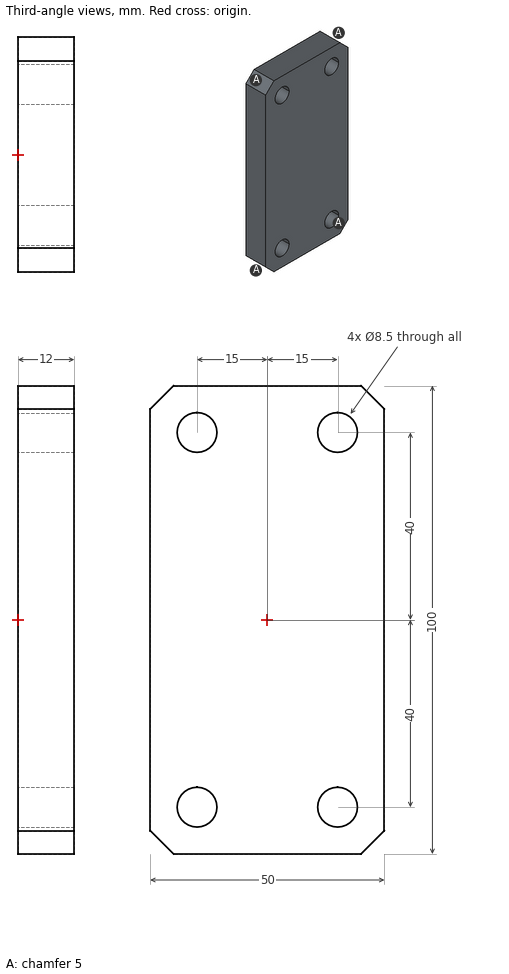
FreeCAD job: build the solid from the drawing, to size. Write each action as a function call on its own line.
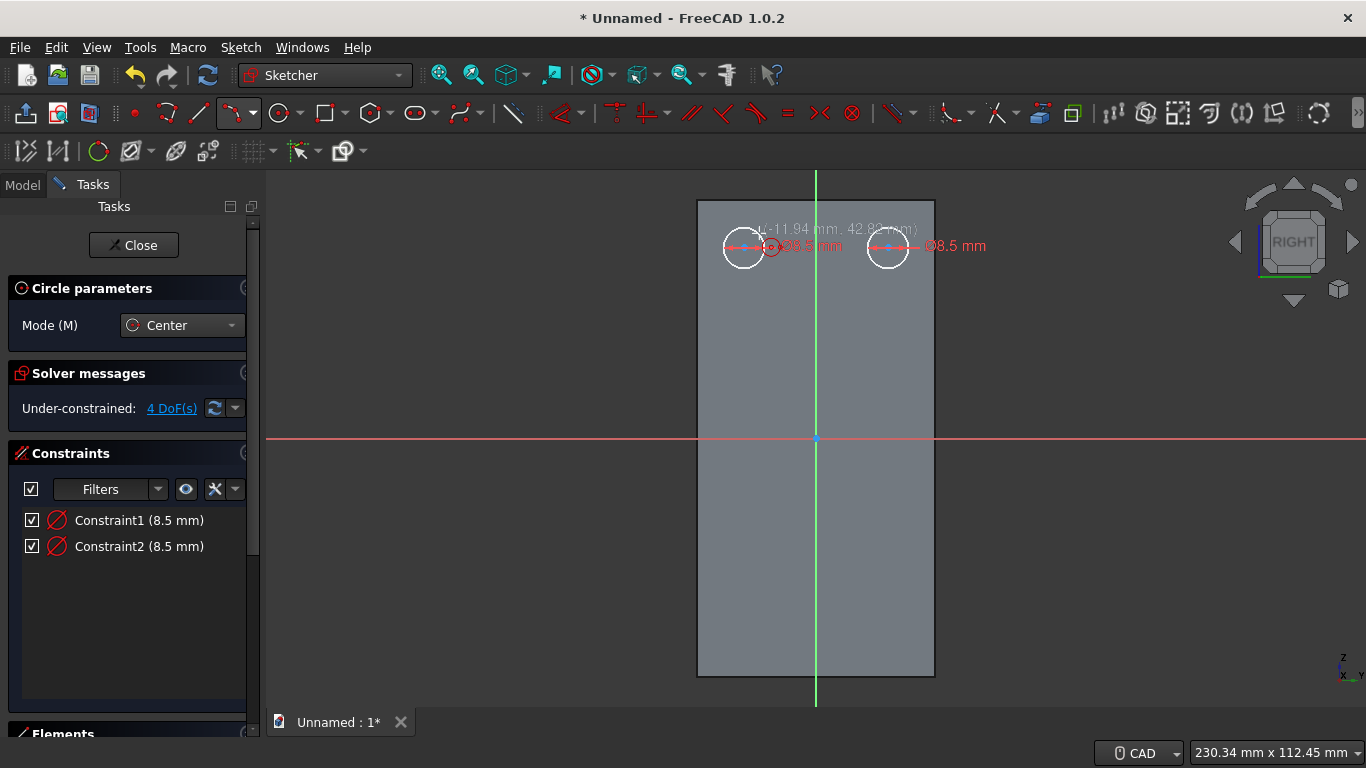
click(888, 630)
move(902, 615)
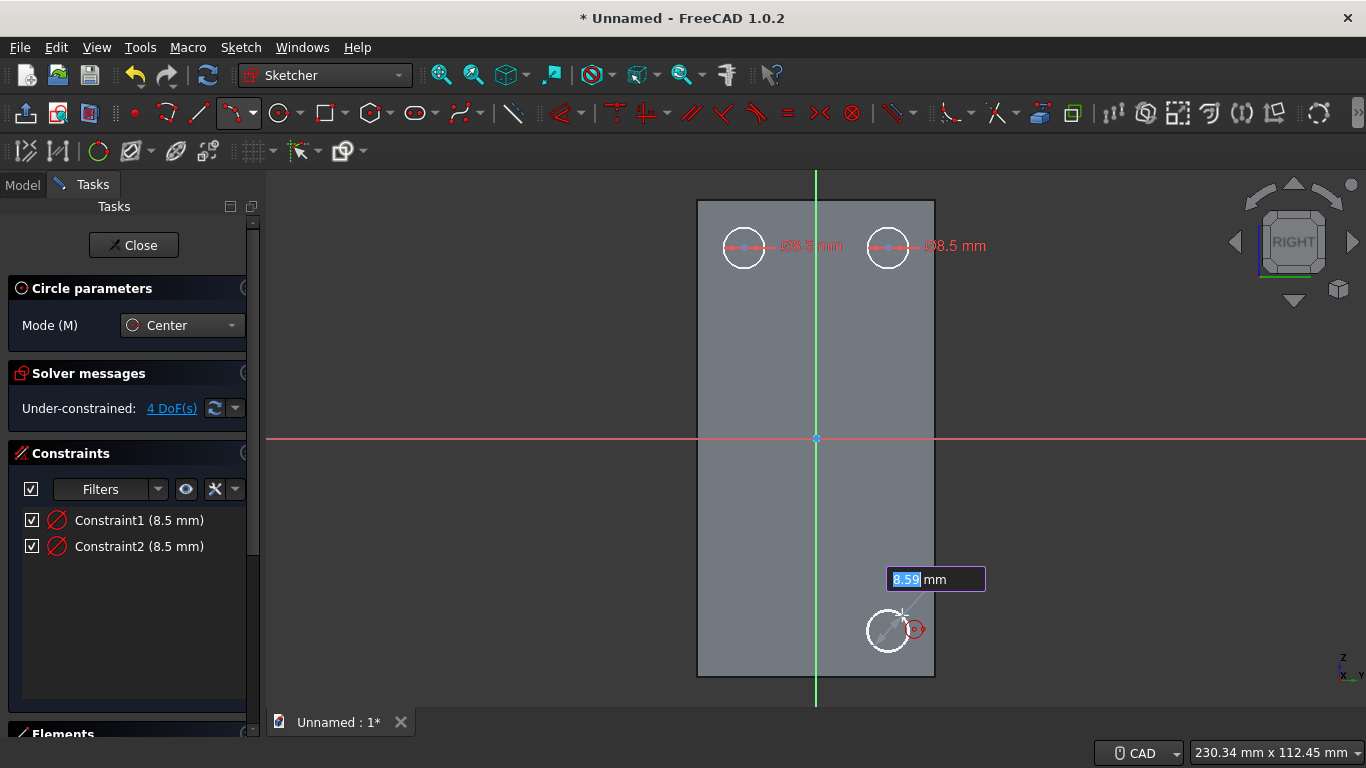
text(8.5)
key(Return)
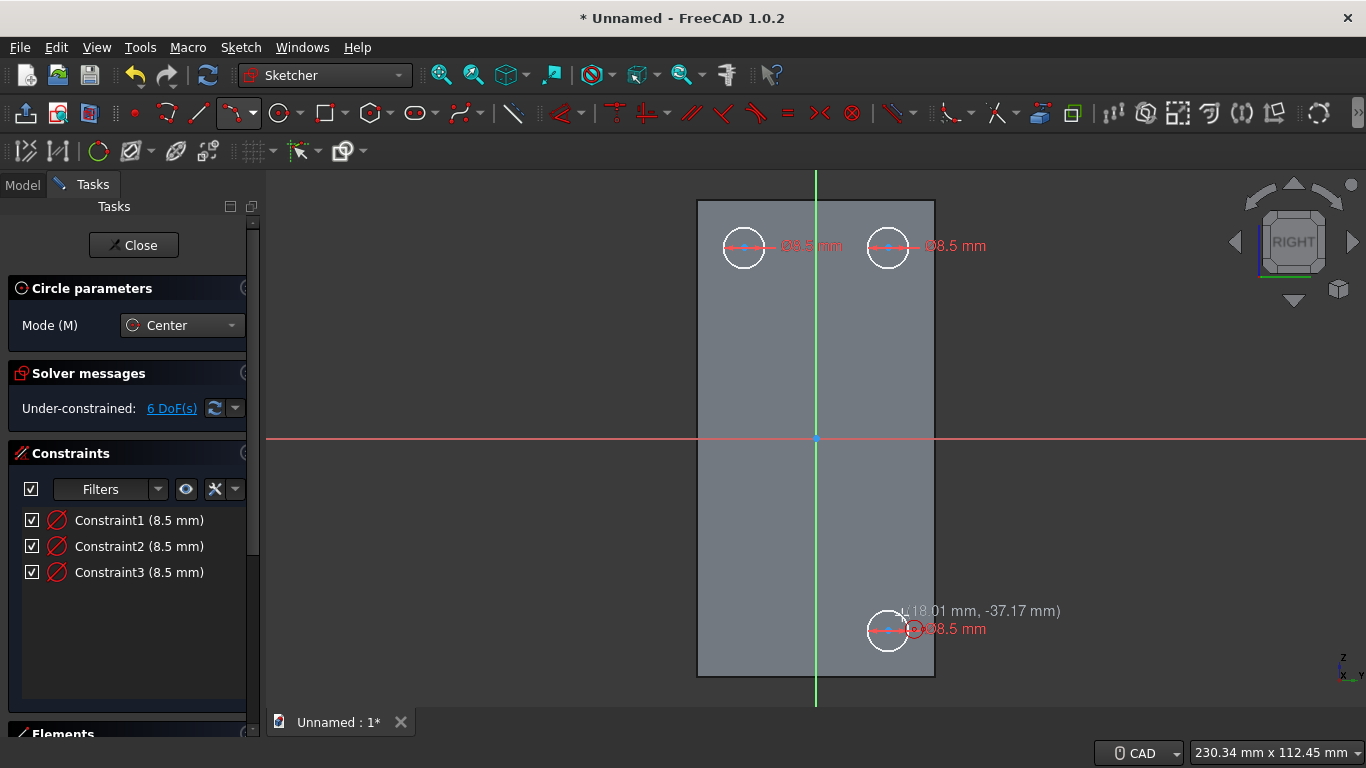
click(744, 630)
move(759, 615)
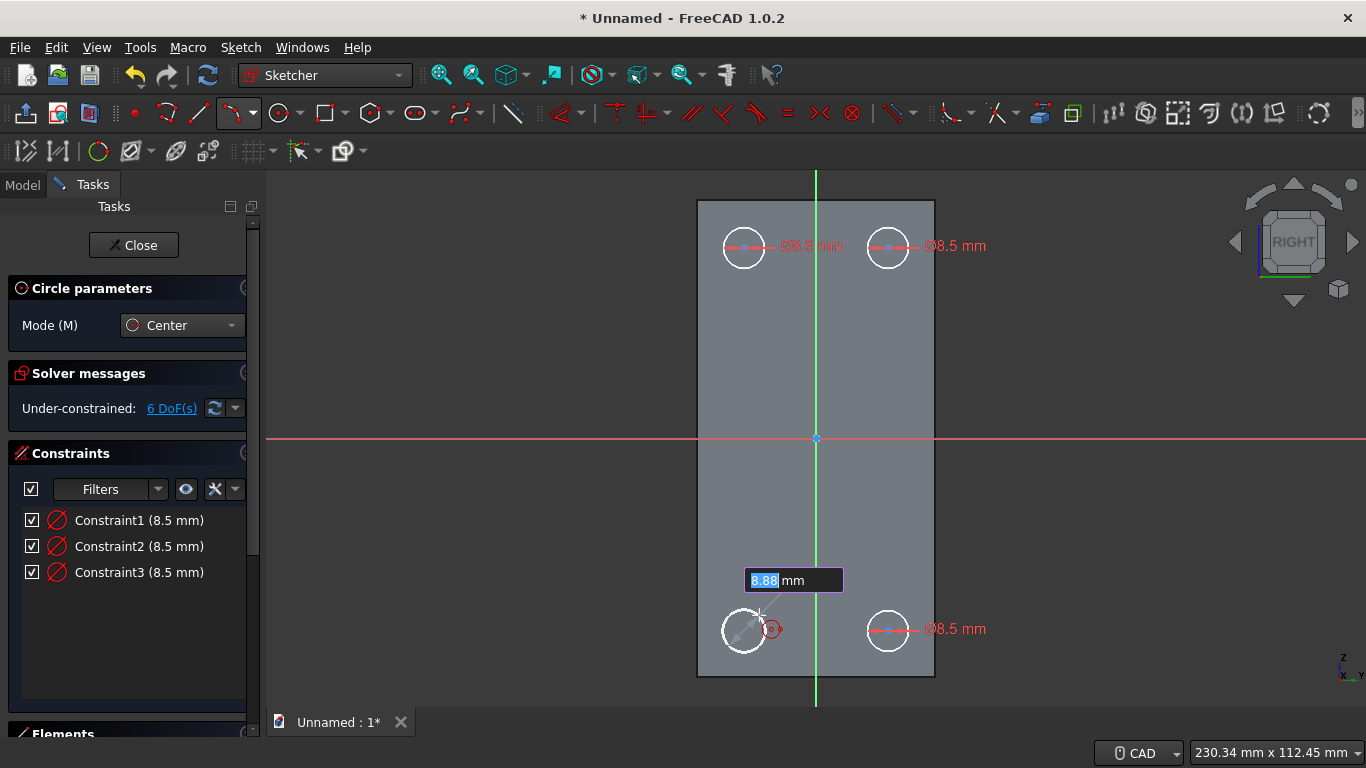
text(8.5)
key(Return)
key(Escape)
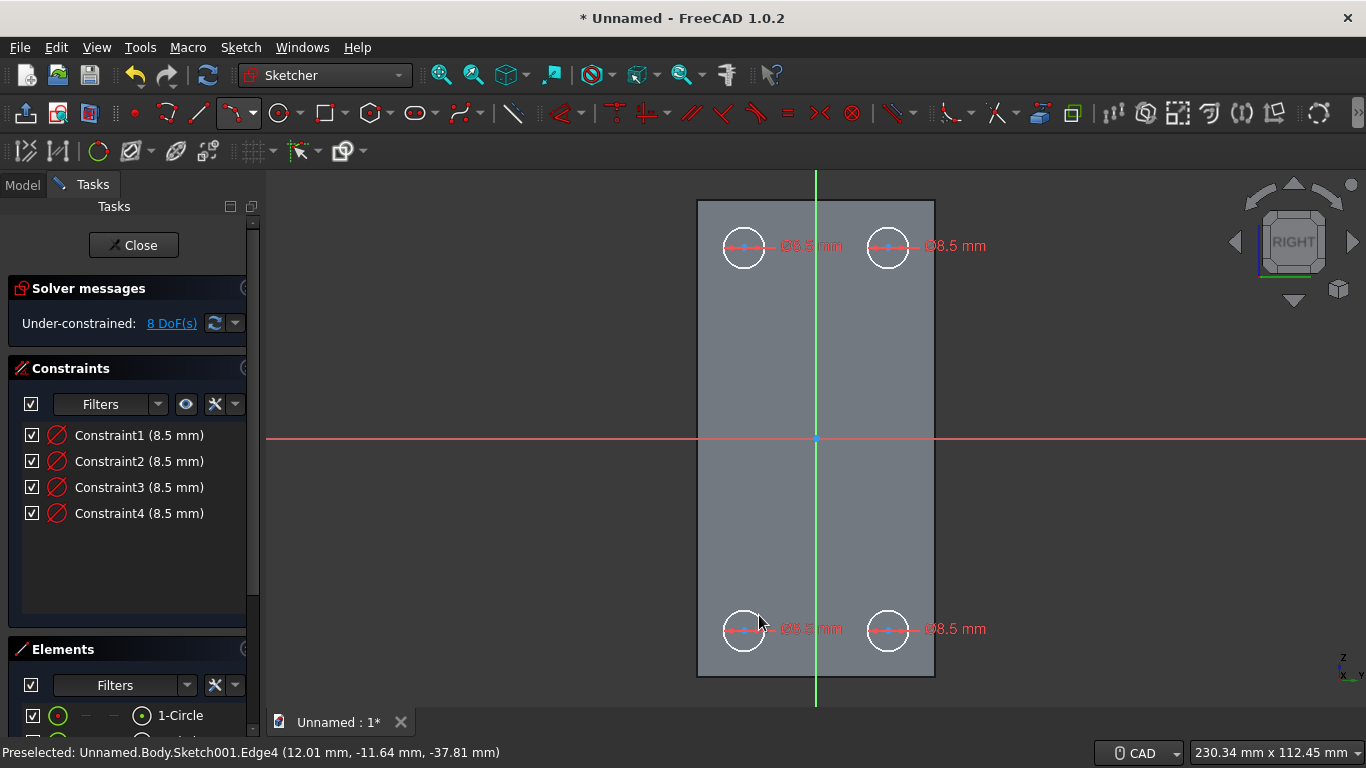
click(888, 248)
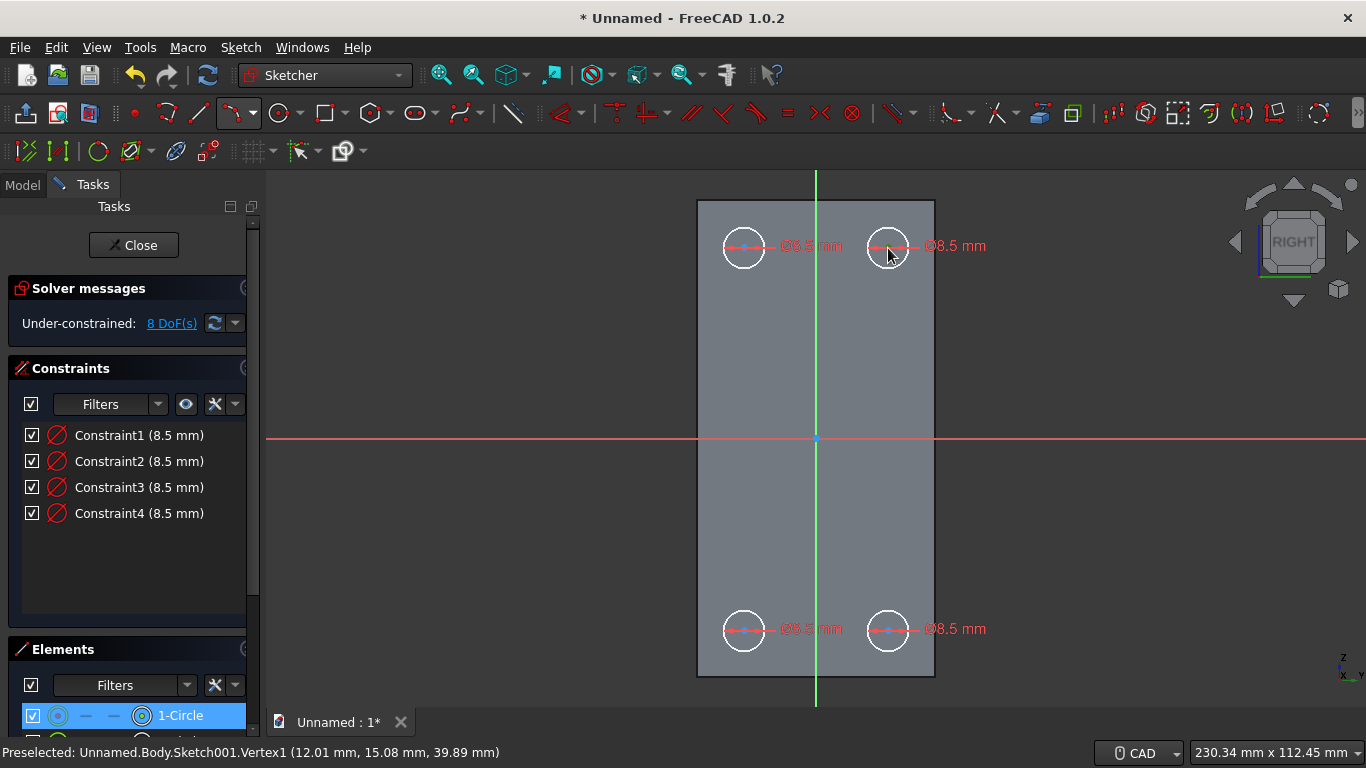
click(744, 248)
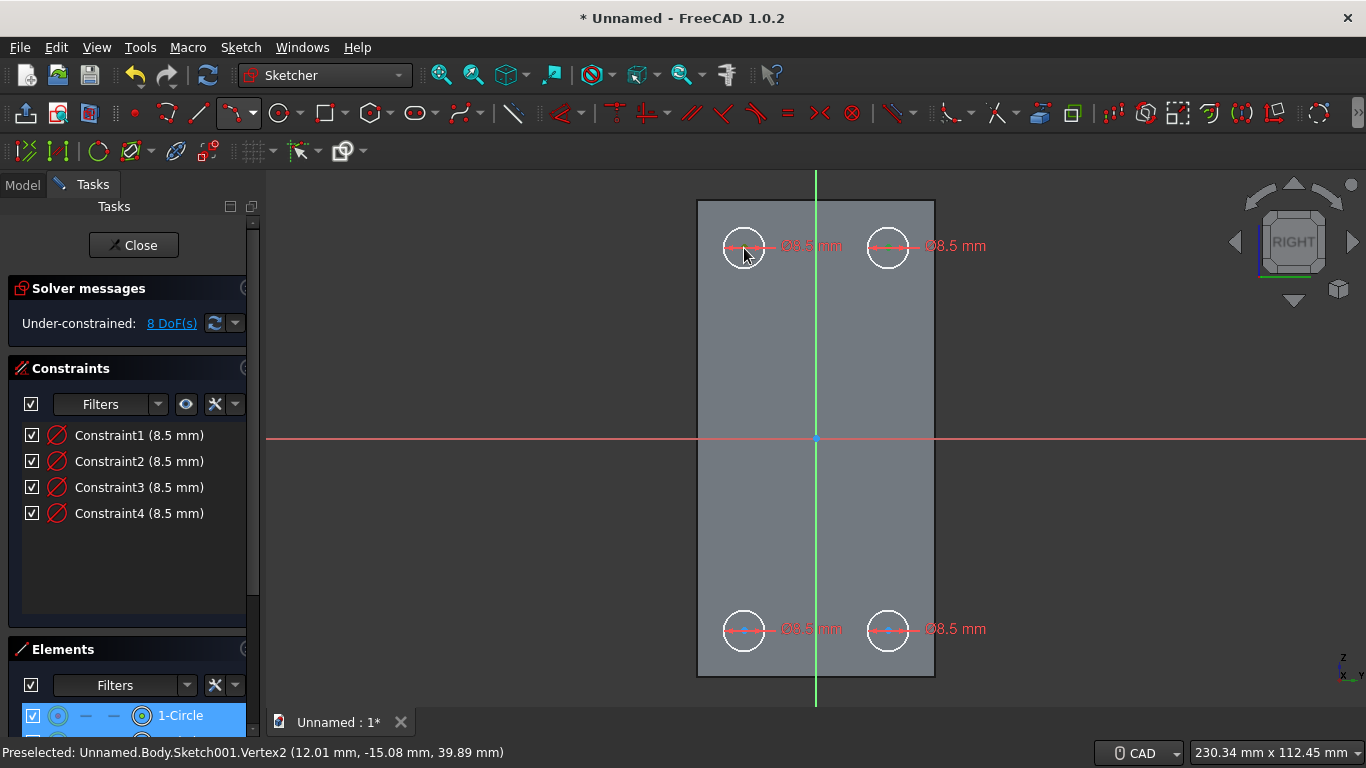
click(670, 114)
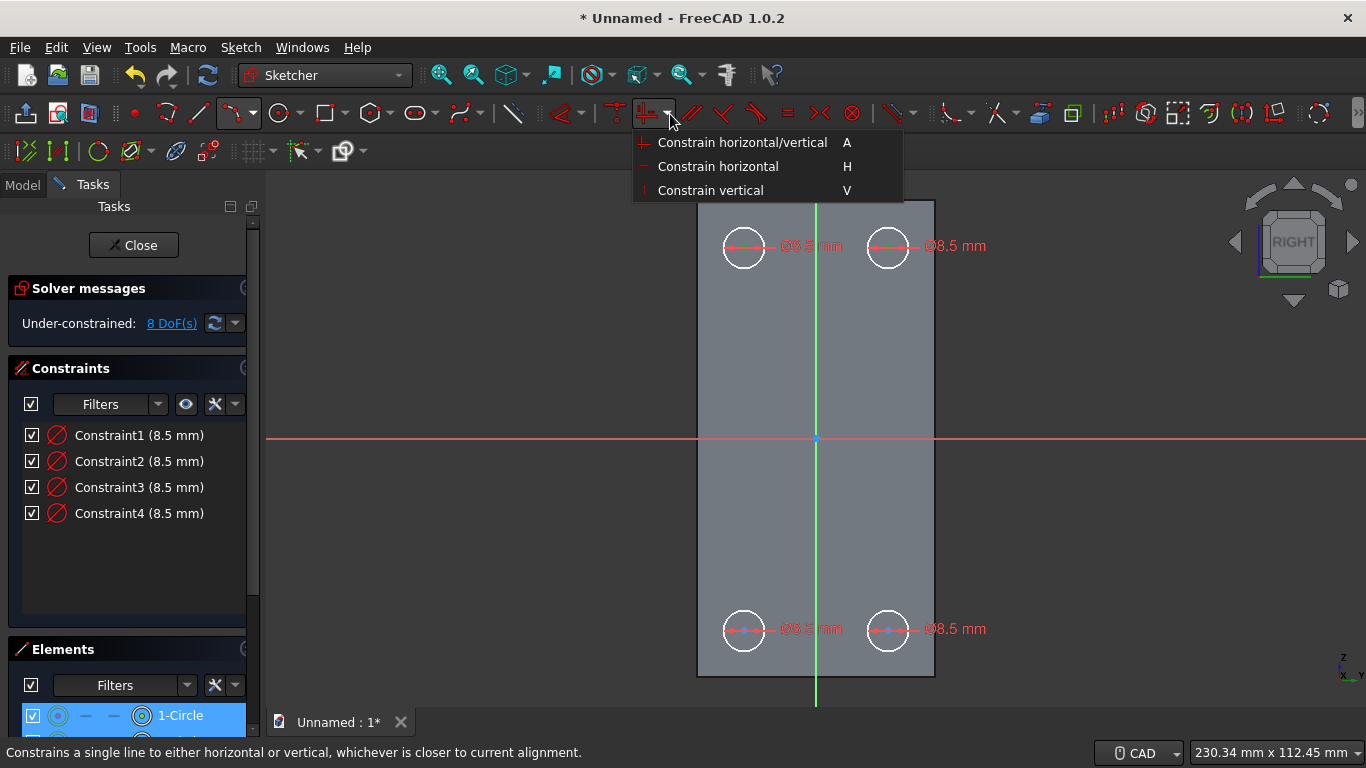
click(768, 166)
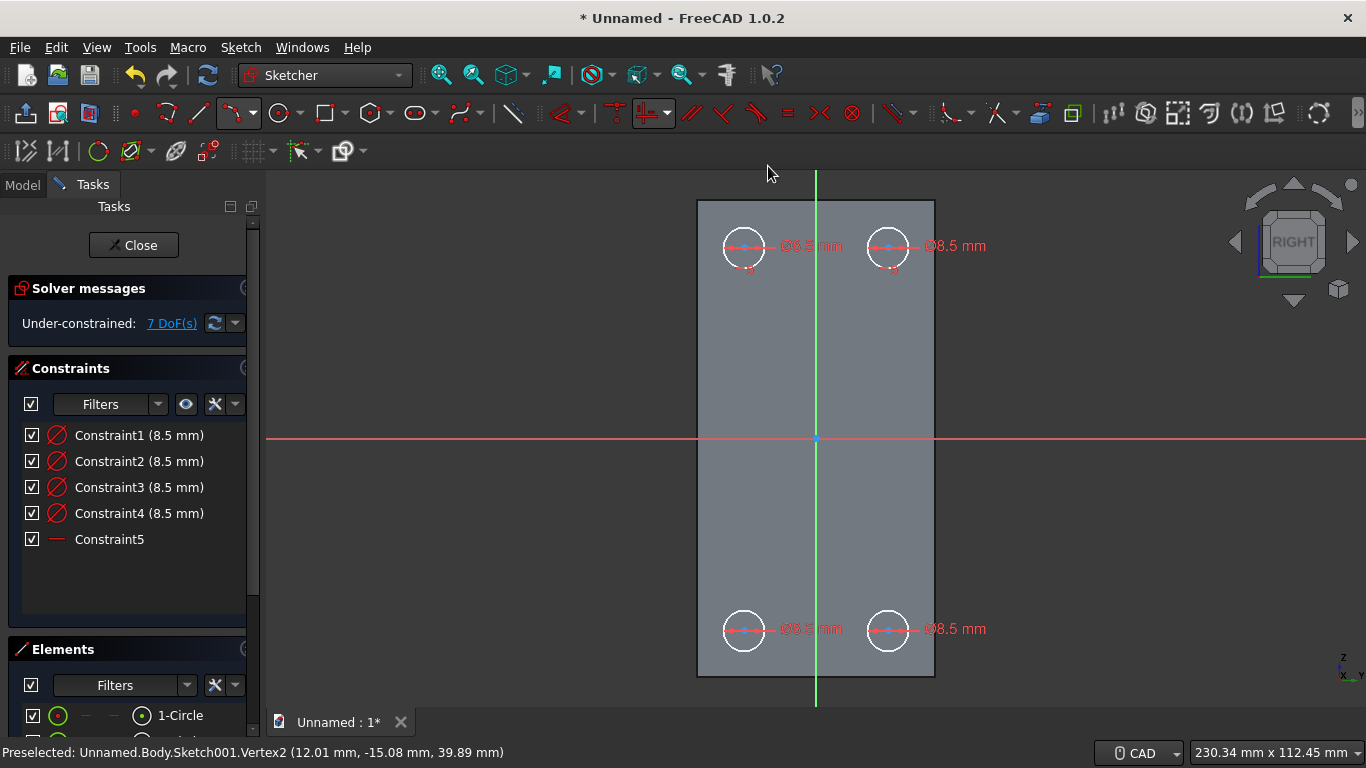
click(888, 248)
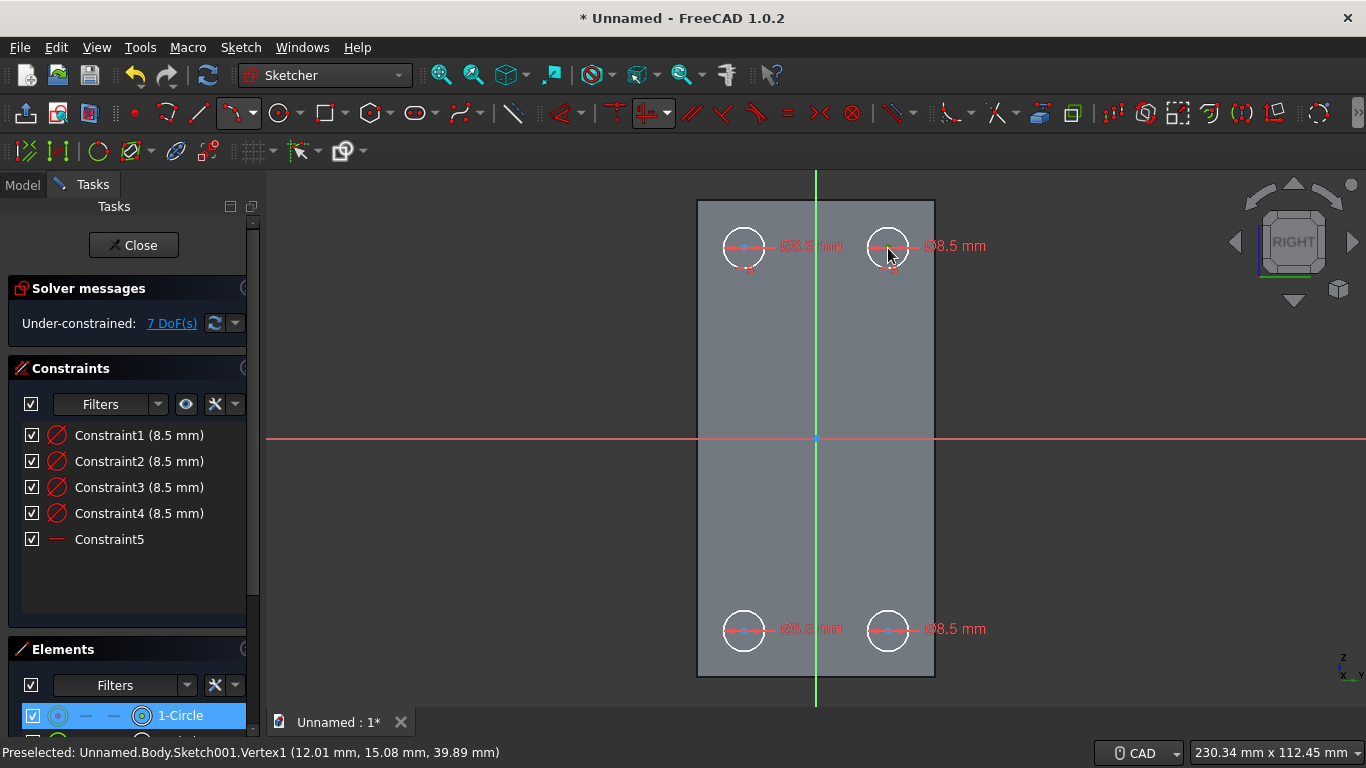
click(888, 631)